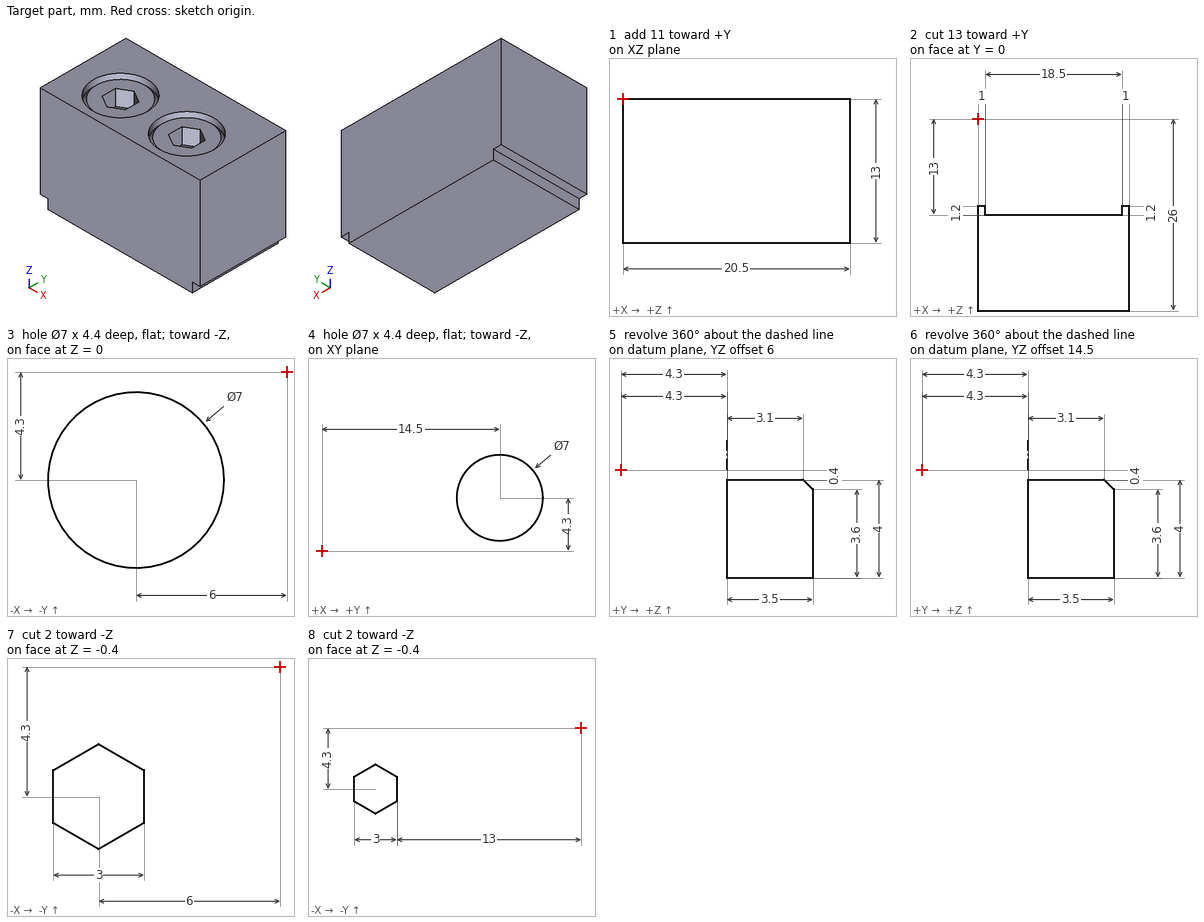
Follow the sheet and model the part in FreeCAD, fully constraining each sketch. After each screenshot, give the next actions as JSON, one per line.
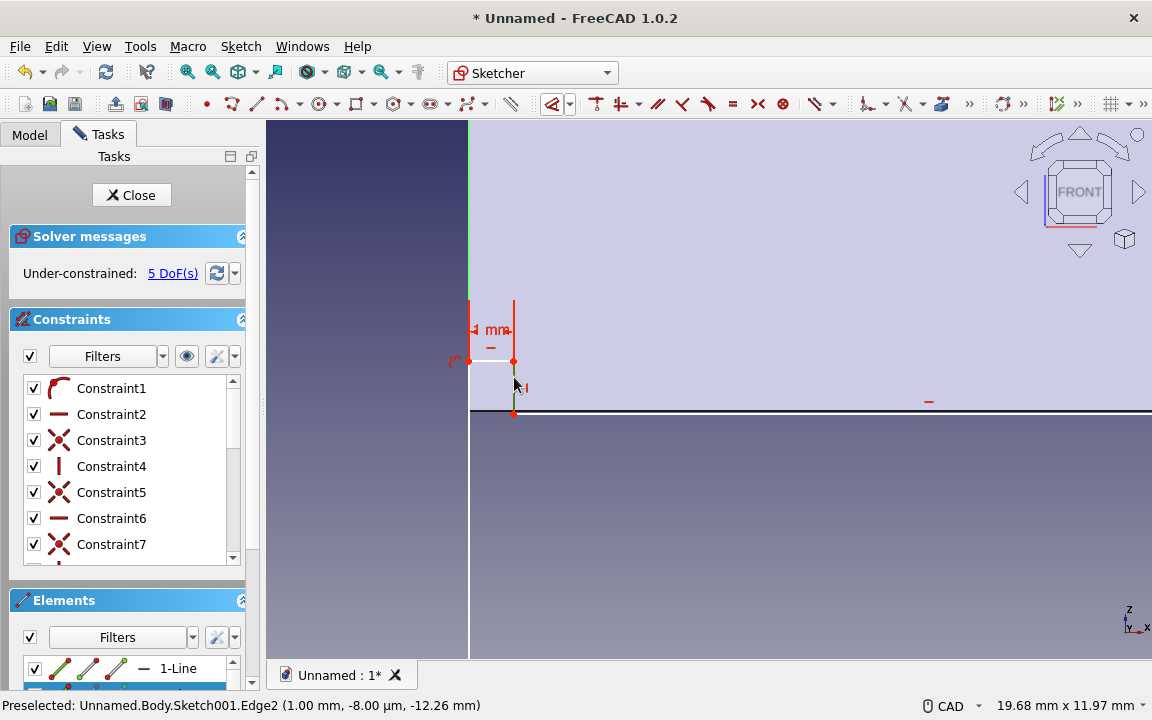
{"action": "left_click", "coordinate": [570, 104]}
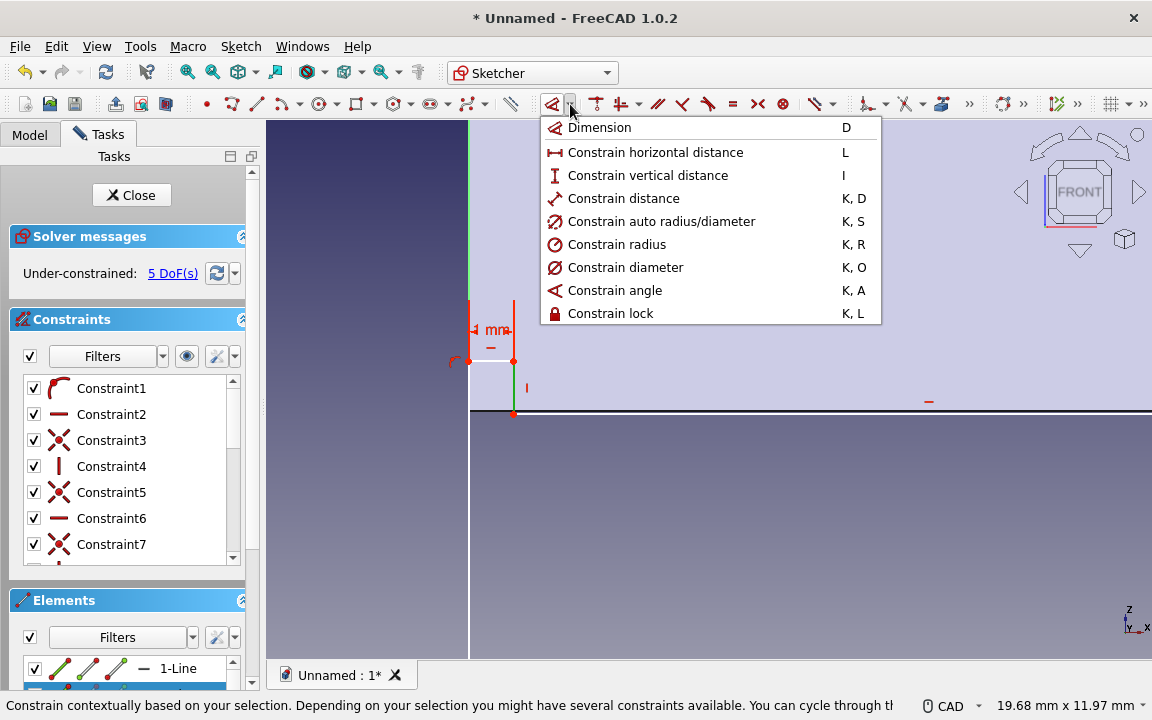
{"action": "left_click", "coordinate": [711, 176]}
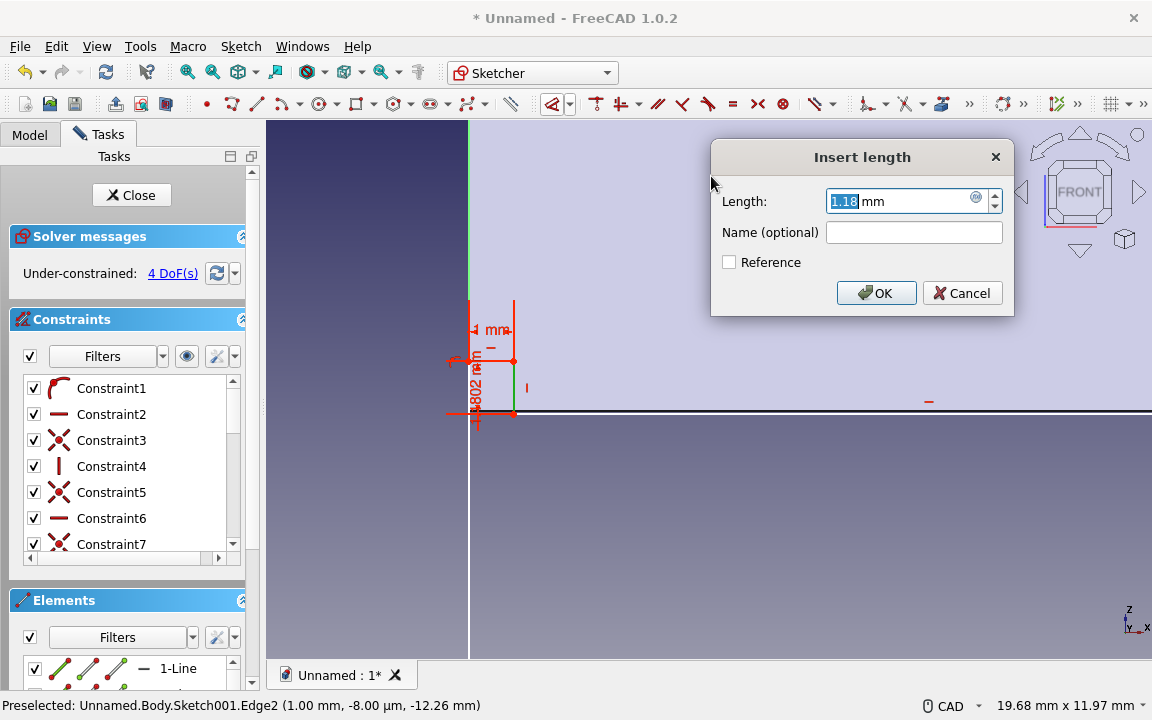
{"action": "type", "text": "1.2"}
{"action": "key", "text": "Return"}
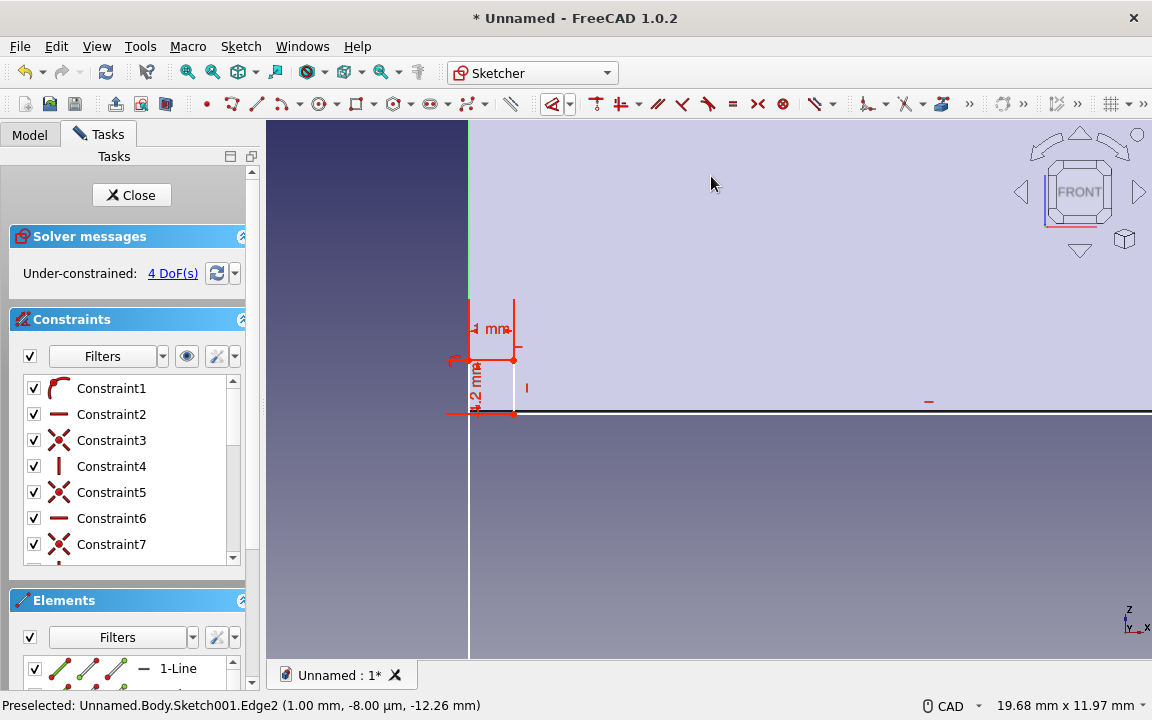
{"action": "scroll", "coordinate": [516, 380], "scroll_direction": "down", "scroll_amount": 6}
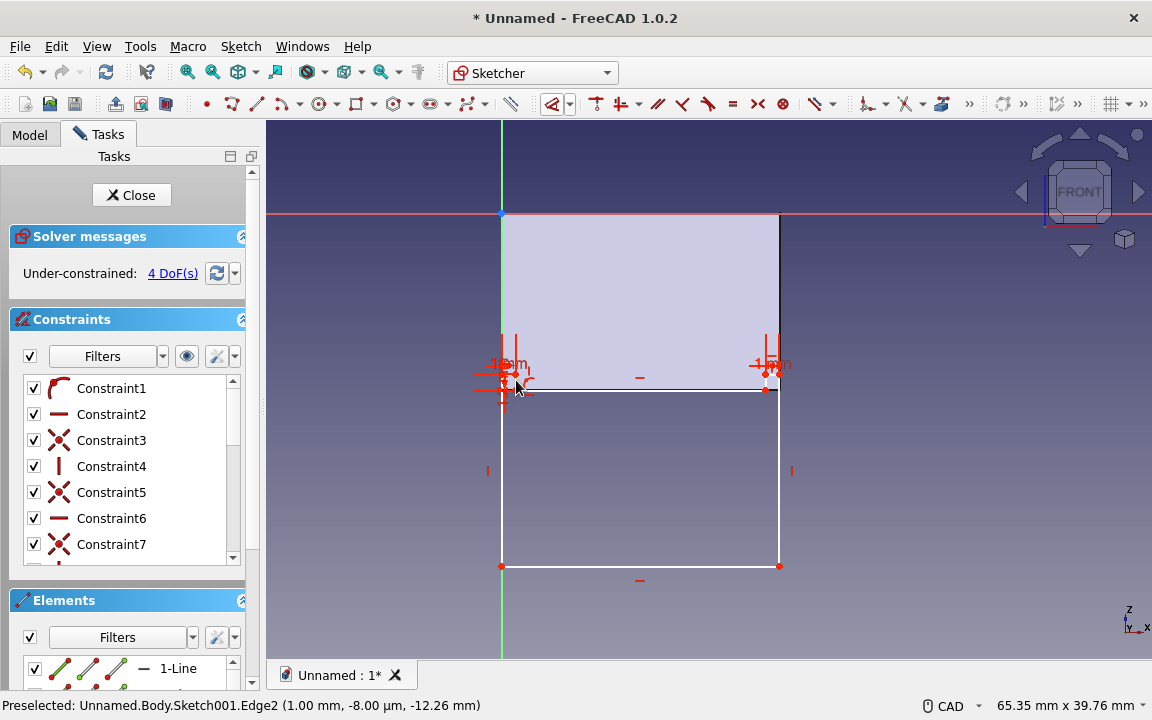
{"action": "scroll", "coordinate": [766, 386], "scroll_direction": "up", "scroll_amount": 6}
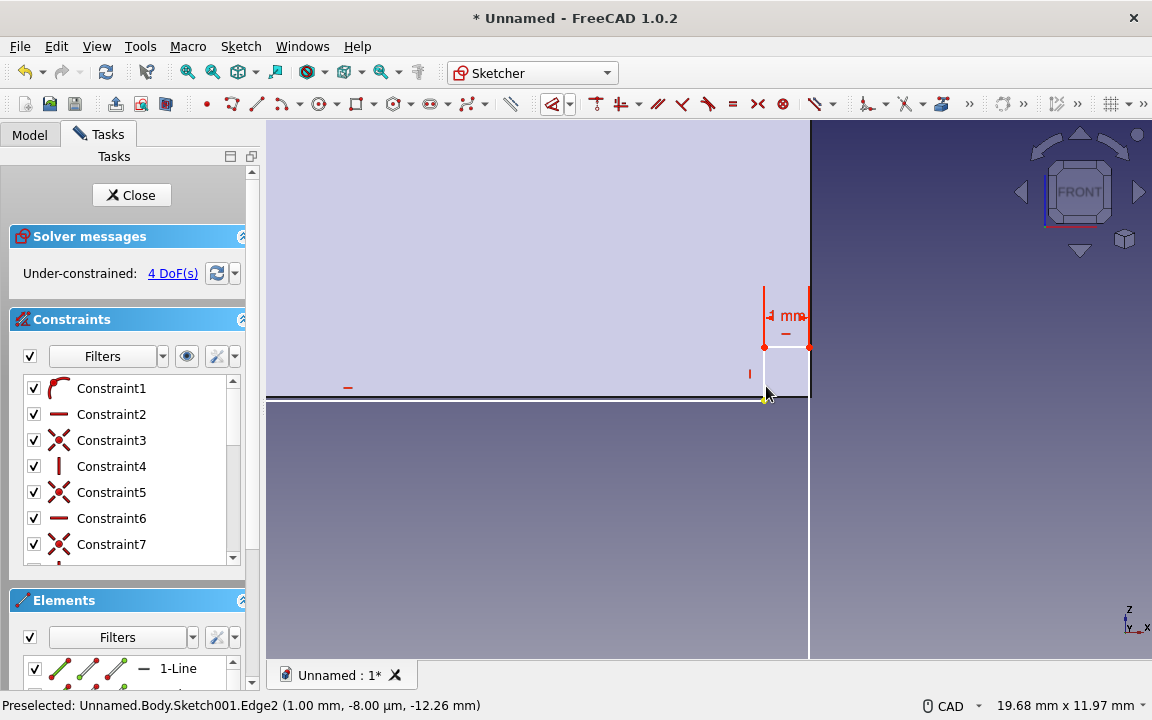
{"action": "left_click", "coordinate": [764, 385]}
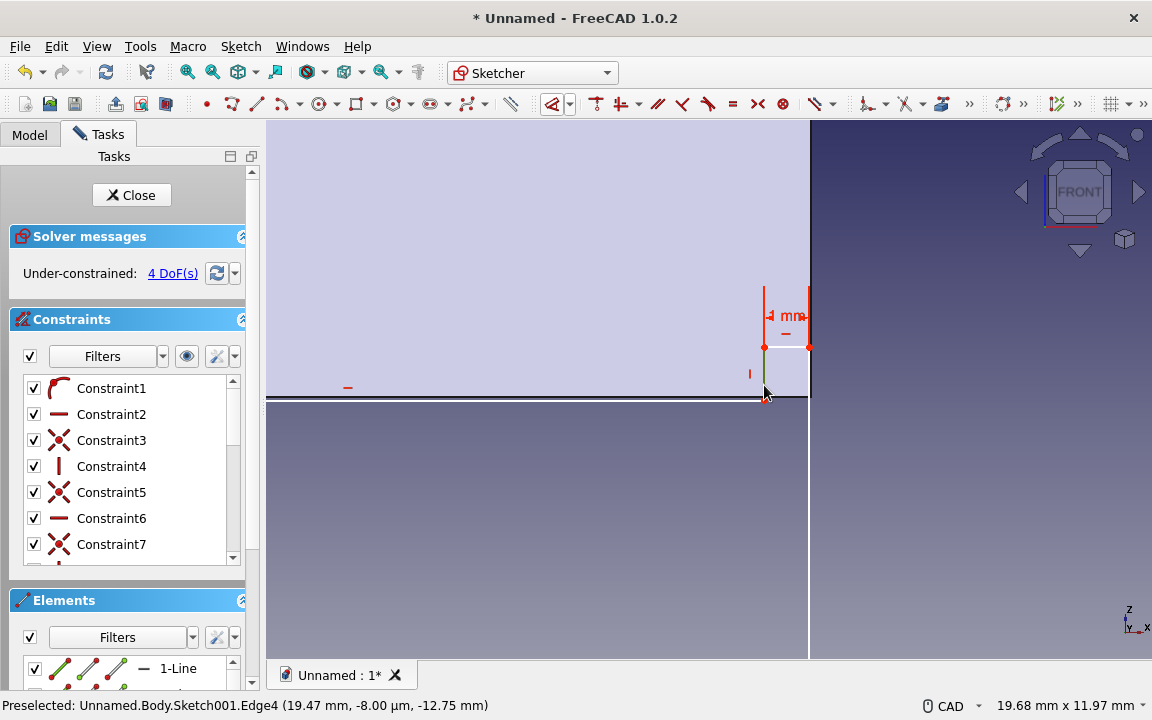
{"action": "key", "text": "i"}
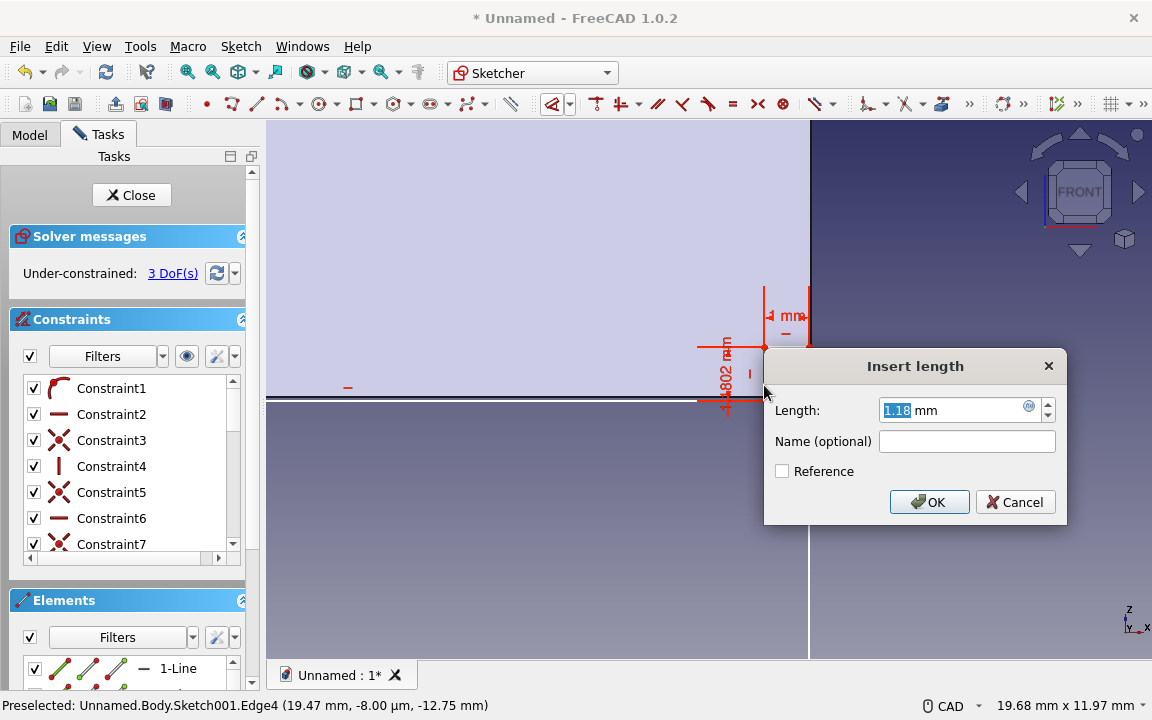
{"action": "type", "text": "1.2"}
{"action": "key", "text": "Return"}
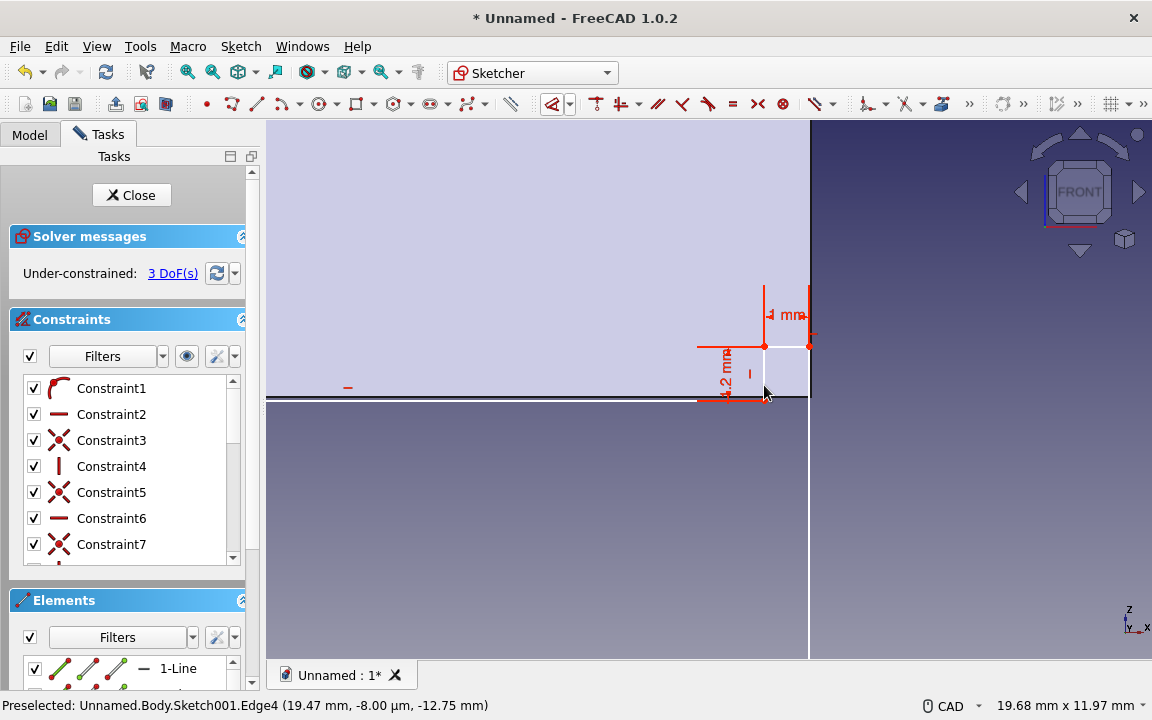
{"action": "scroll", "coordinate": [766, 386], "scroll_direction": "down", "scroll_amount": 6}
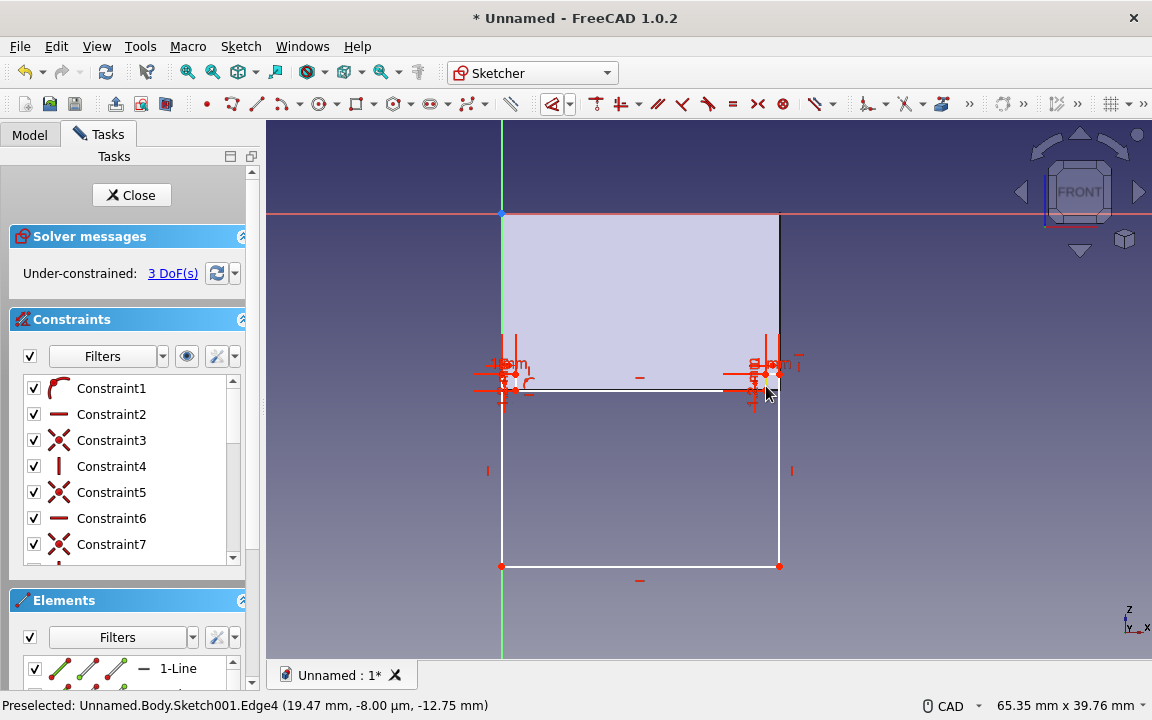
{"action": "left_click", "coordinate": [516, 391]}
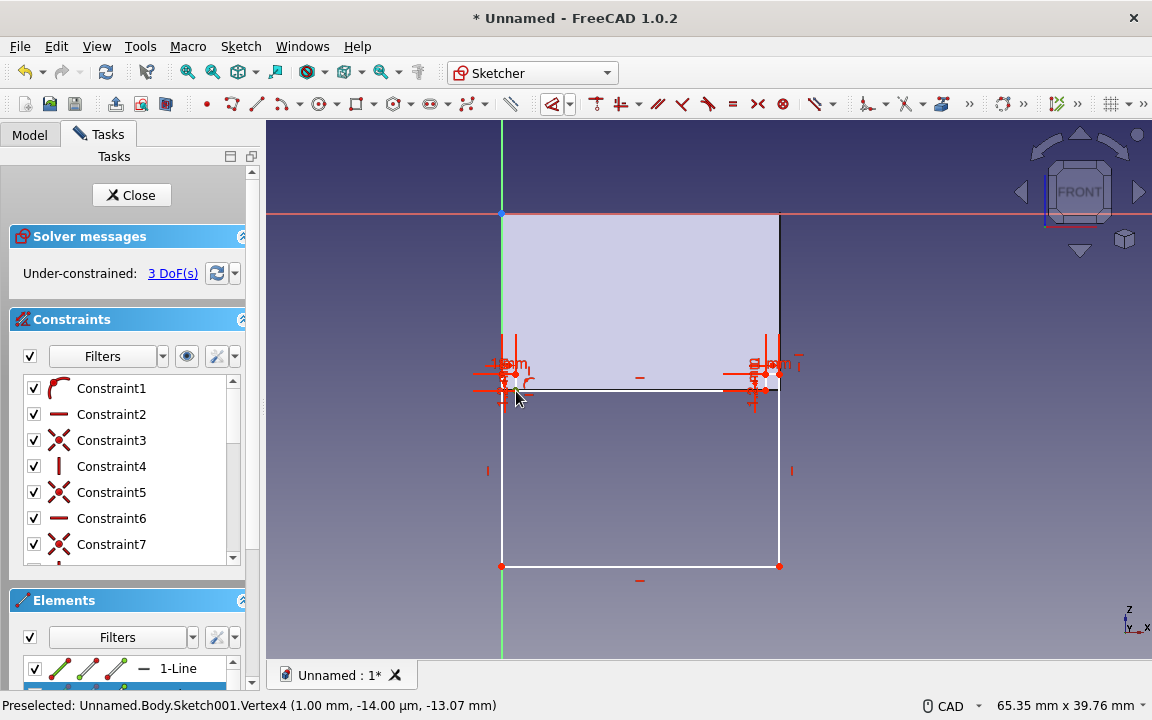
{"action": "key", "text": "i"}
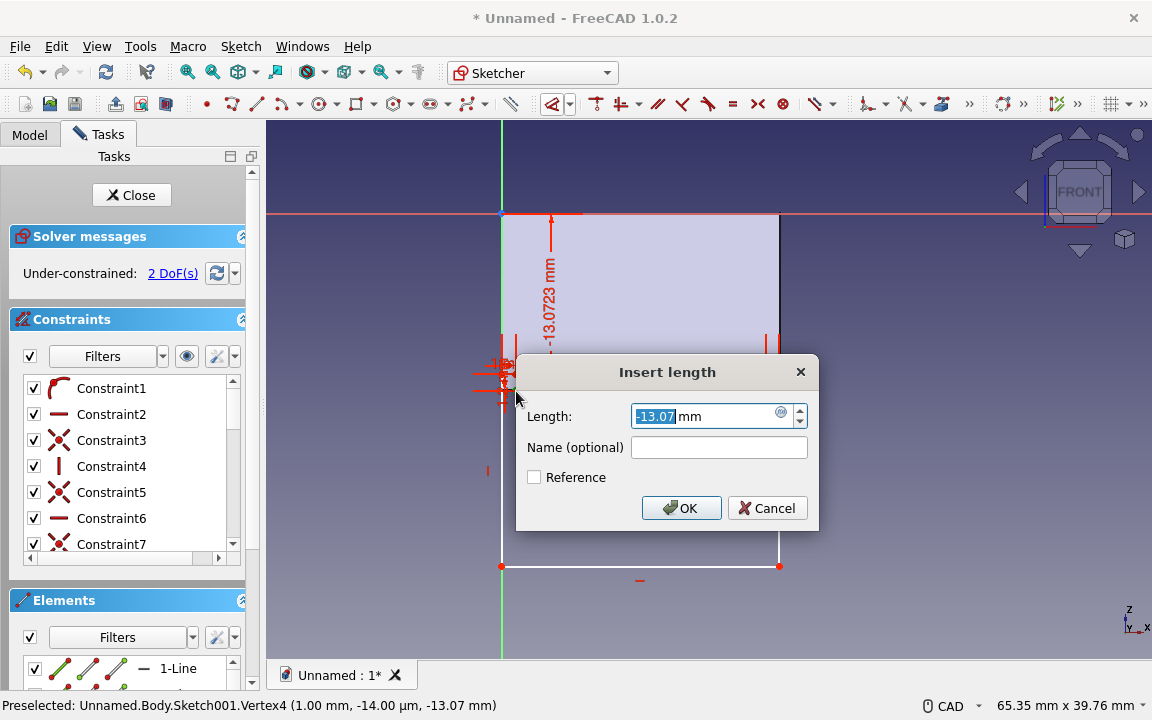
{"action": "type", "text": "-13"}
{"action": "key", "text": "Return"}